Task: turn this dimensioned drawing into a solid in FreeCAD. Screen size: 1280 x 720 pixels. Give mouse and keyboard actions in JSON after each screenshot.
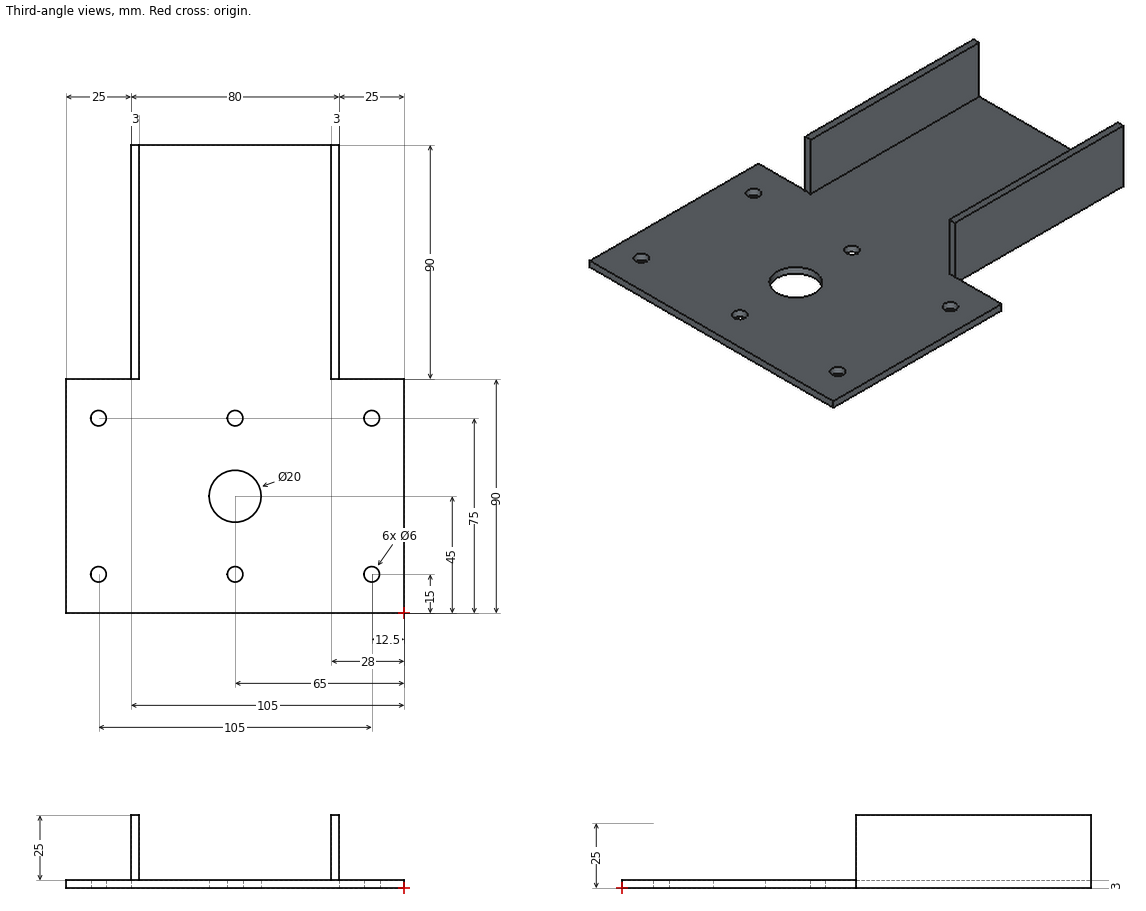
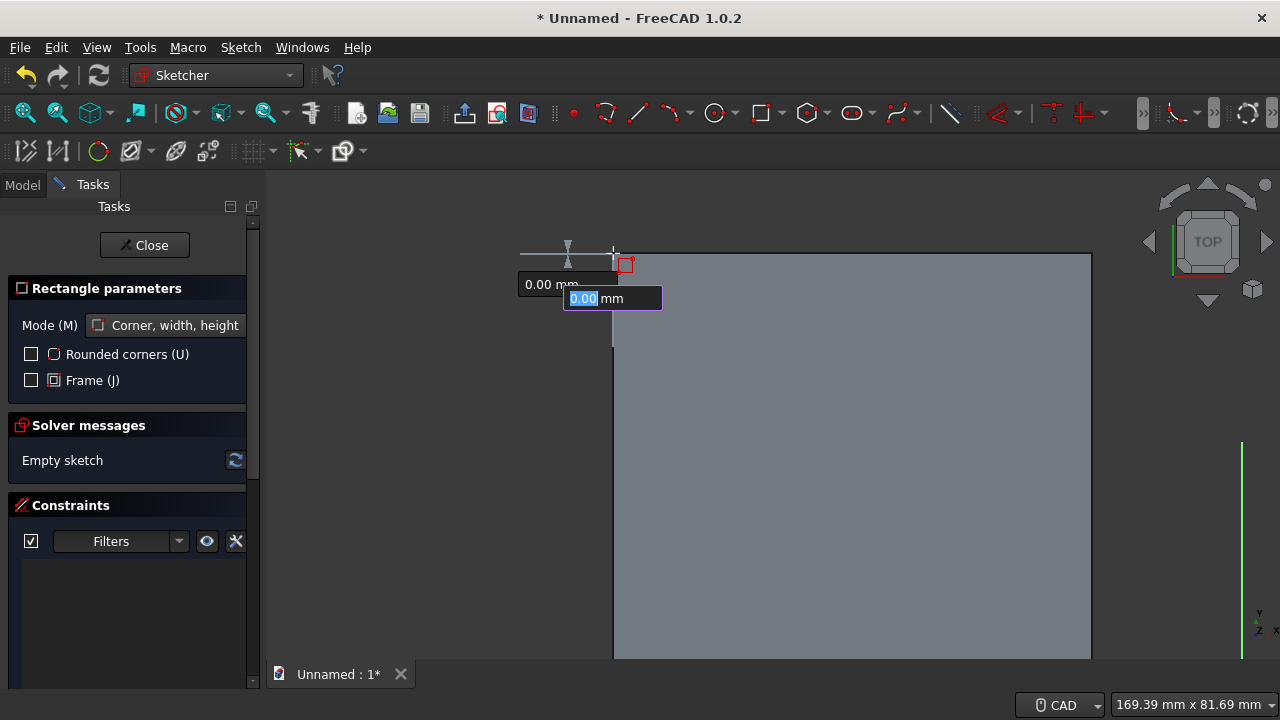
{"action": "scroll", "coordinate": [608, 252], "scroll_direction": "down", "scroll_amount": 6}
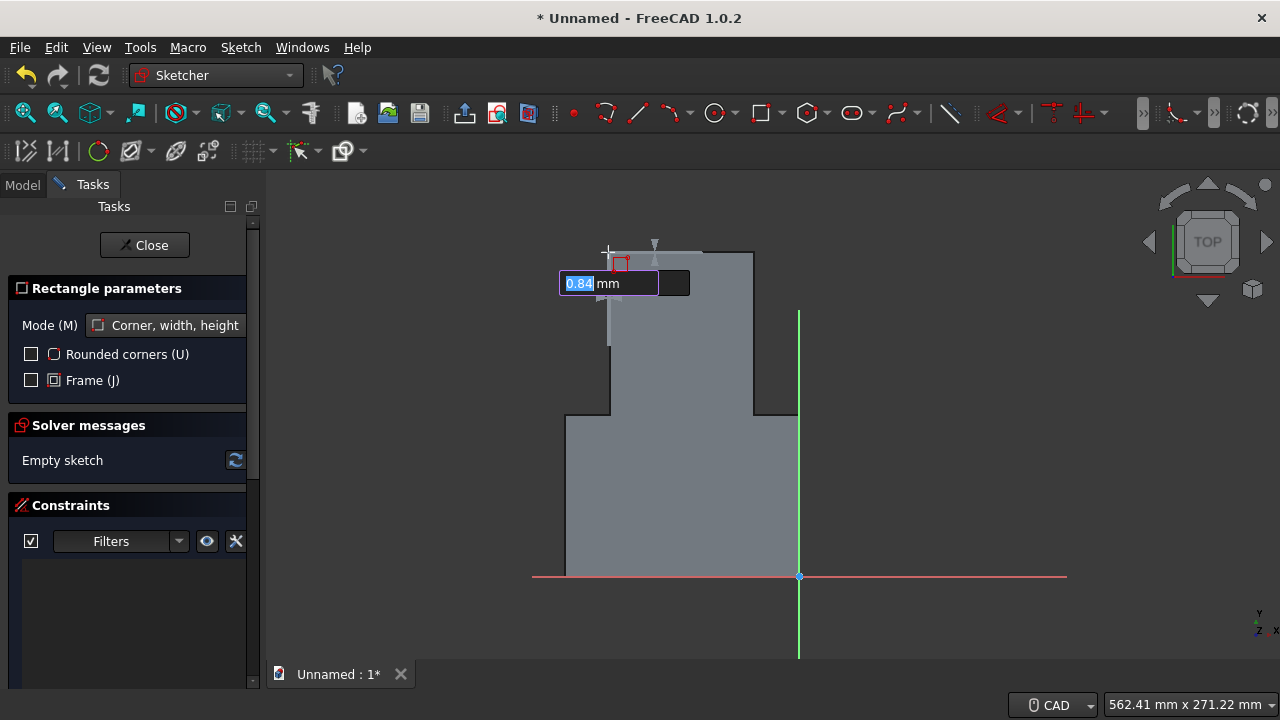
{"action": "left_click", "coordinate": [615, 415]}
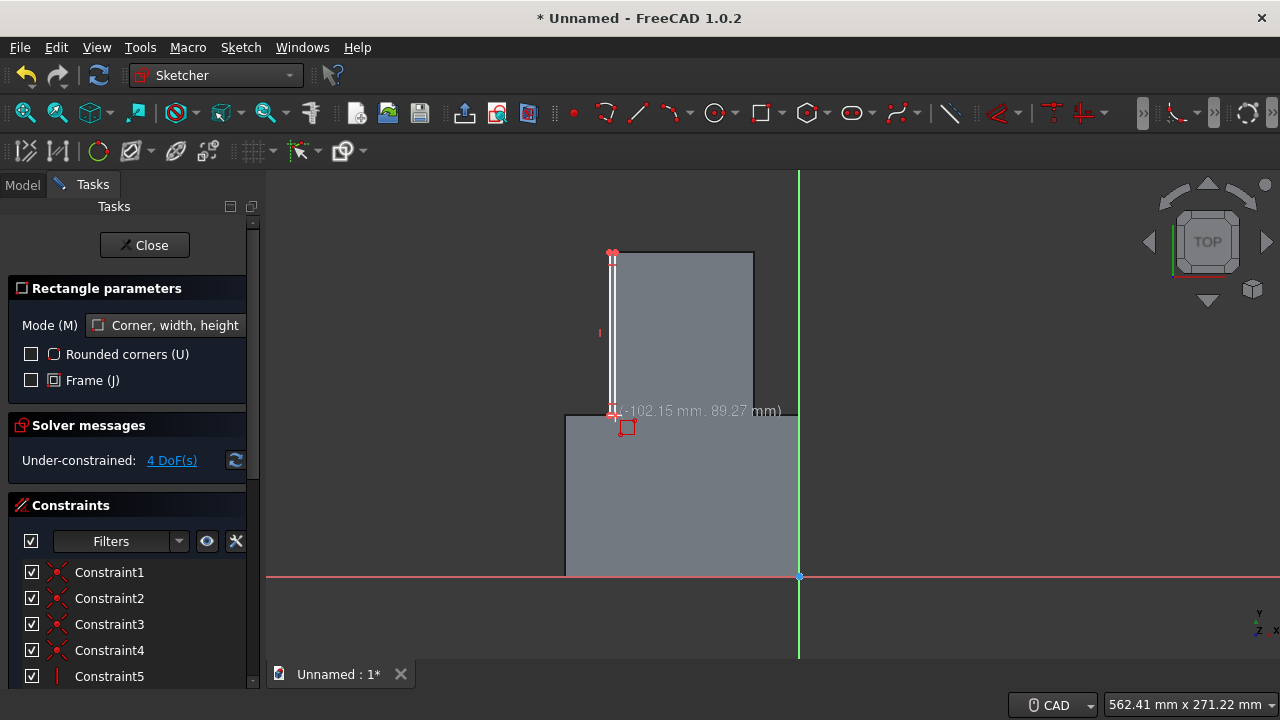
{"action": "scroll", "coordinate": [749, 252], "scroll_direction": "up", "scroll_amount": 6}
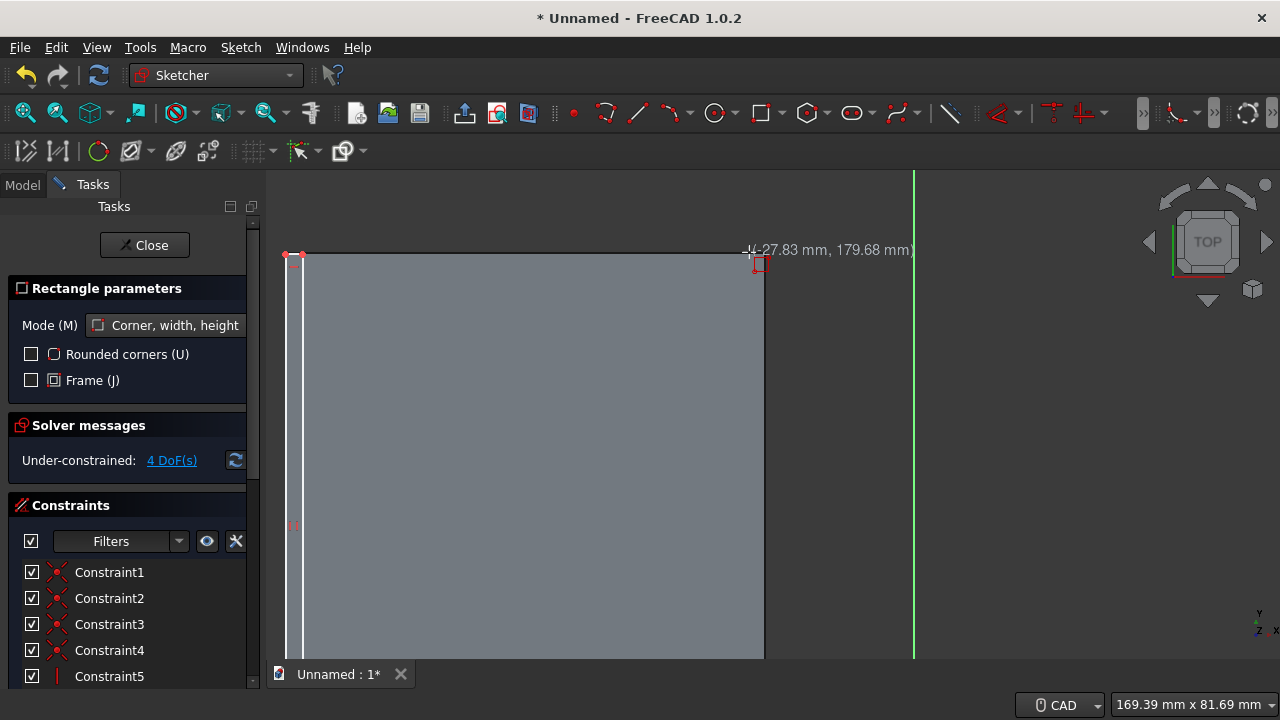
{"action": "left_click", "coordinate": [747, 253]}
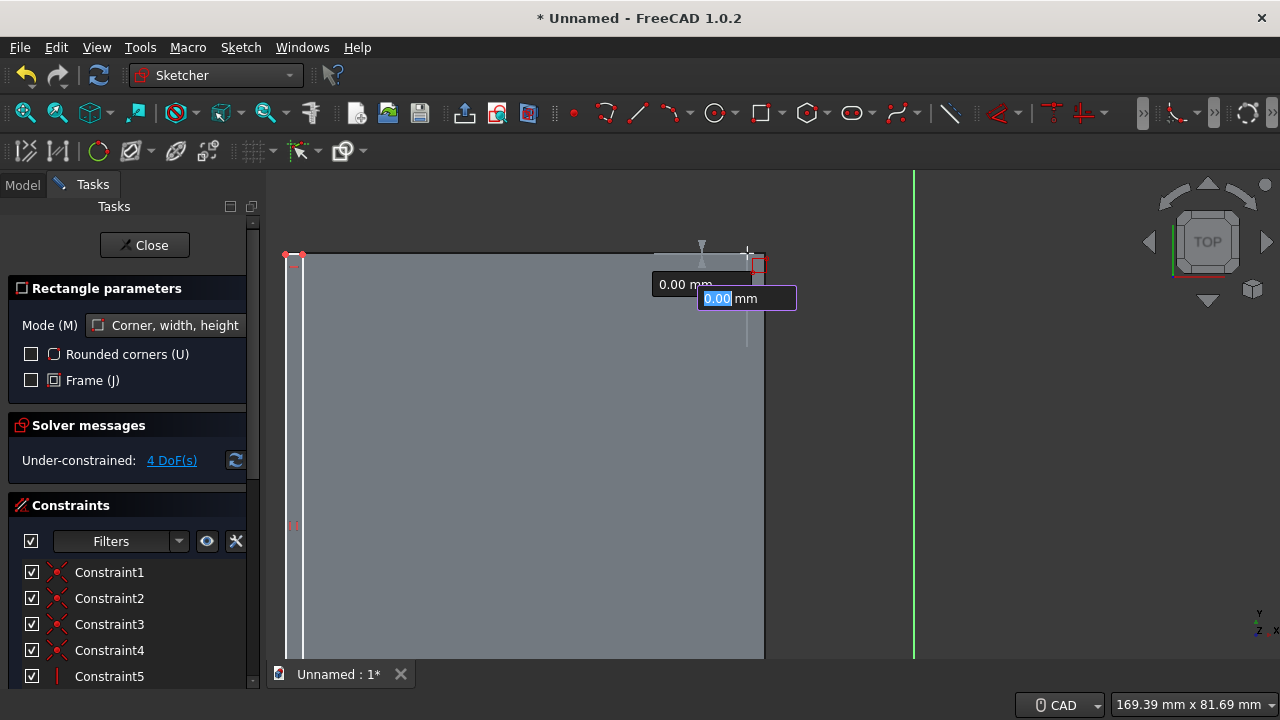
{"action": "scroll", "coordinate": [749, 252], "scroll_direction": "down", "scroll_amount": 6}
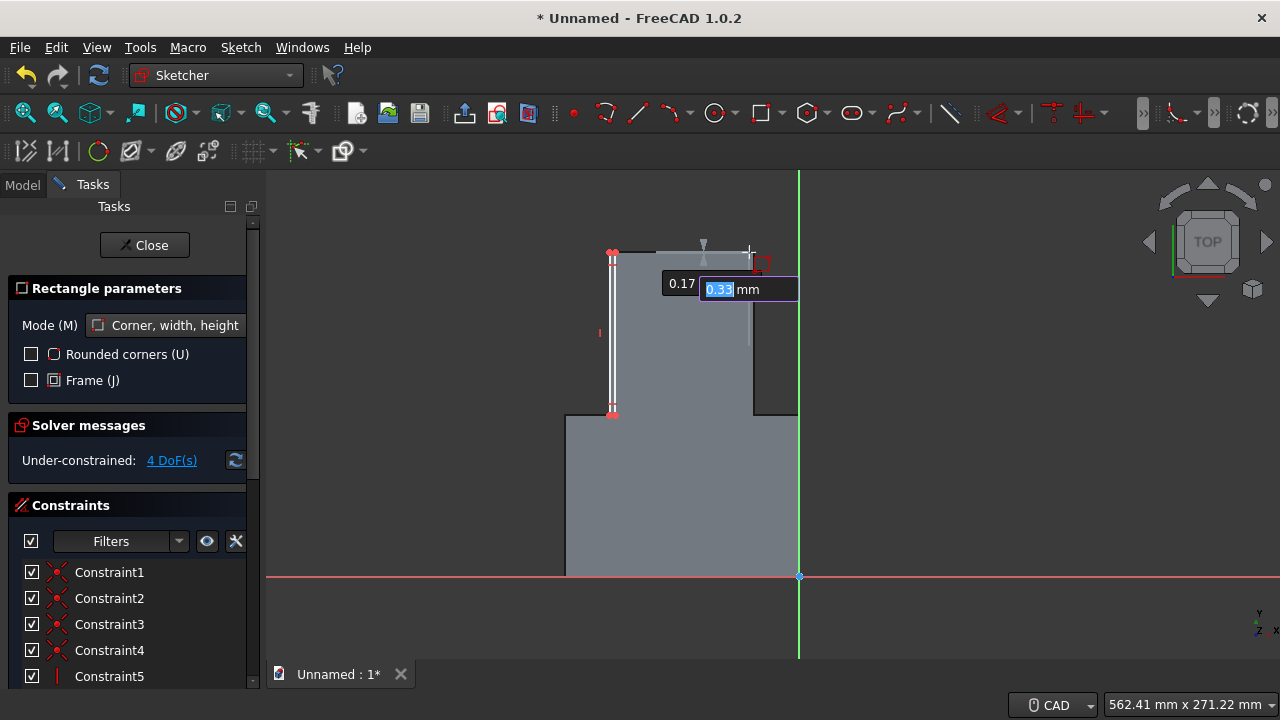
{"action": "left_click", "coordinate": [754, 415]}
{"action": "key", "text": "Escape"}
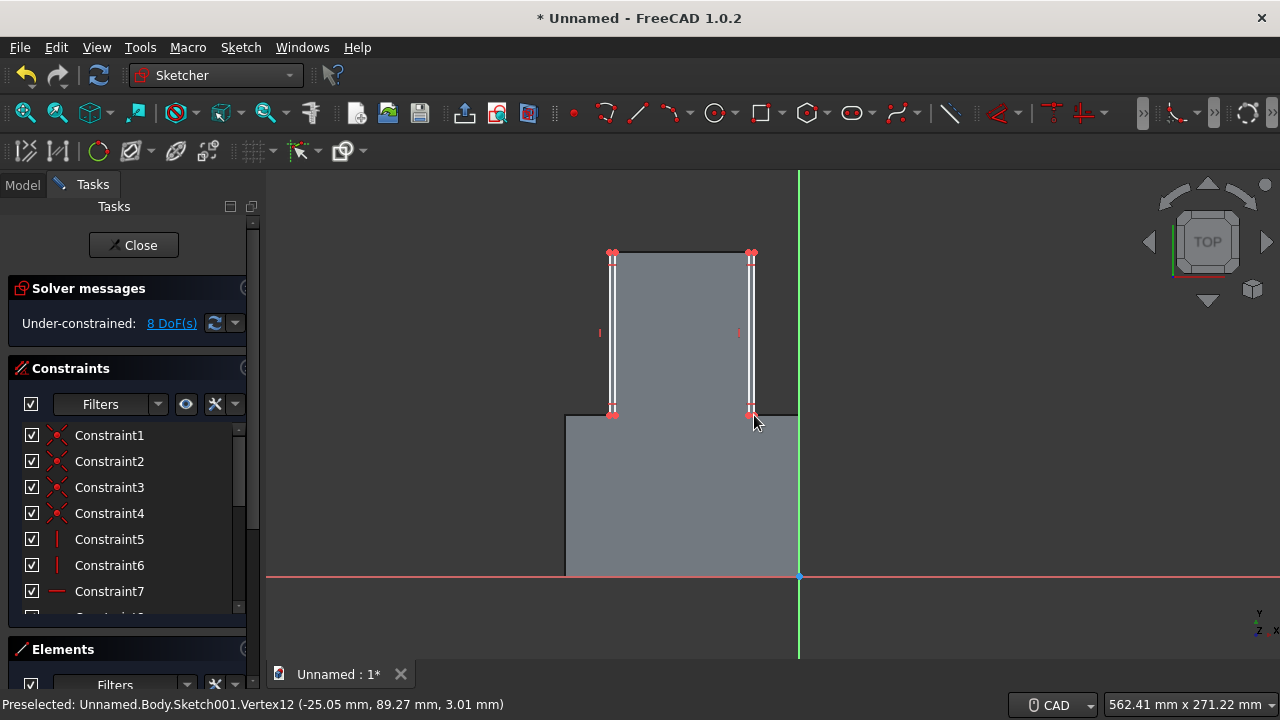
{"action": "left_click", "coordinate": [998, 114]}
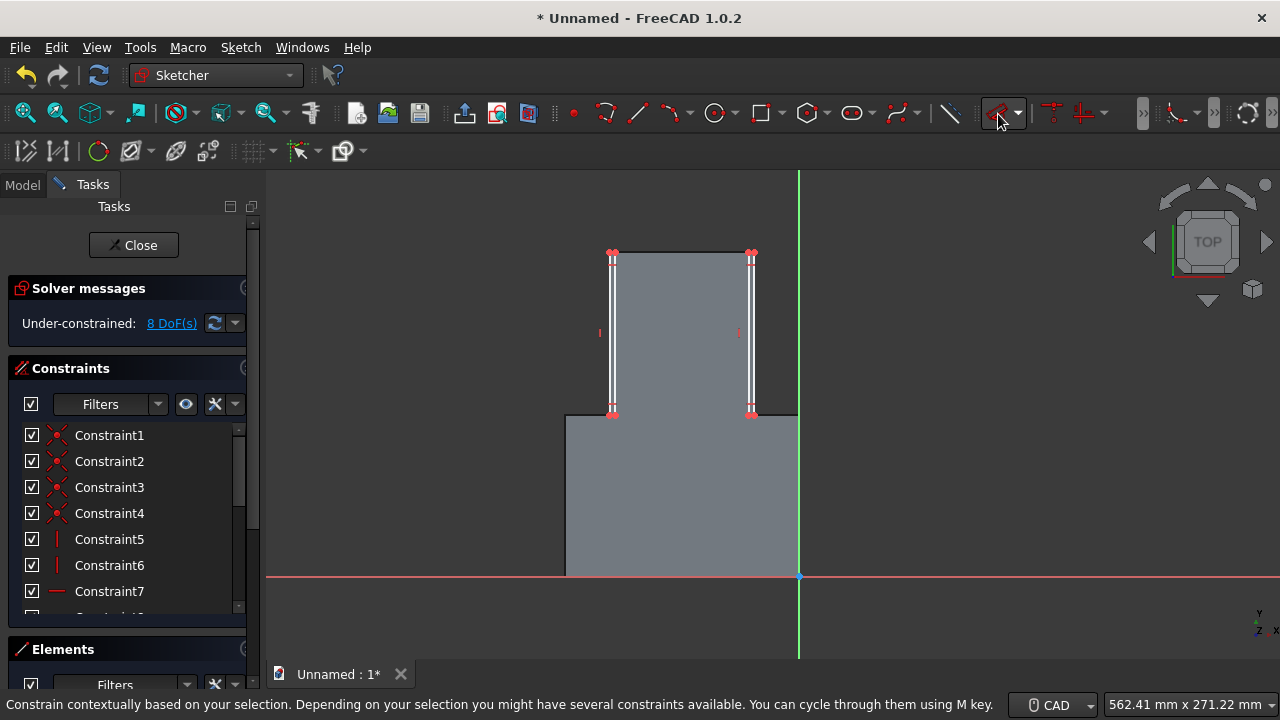
{"action": "scroll", "coordinate": [612, 416], "scroll_direction": "up", "scroll_amount": 10}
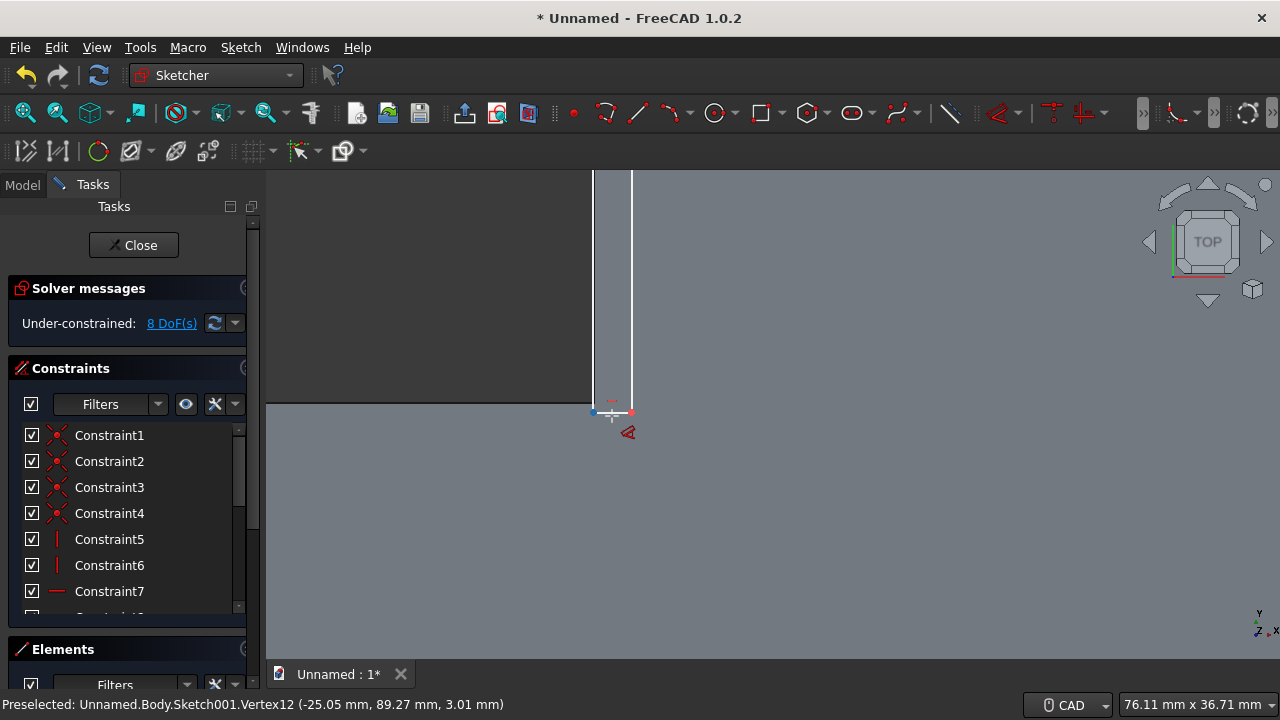
{"action": "left_click", "coordinate": [613, 413]}
{"action": "left_click", "coordinate": [613, 447]}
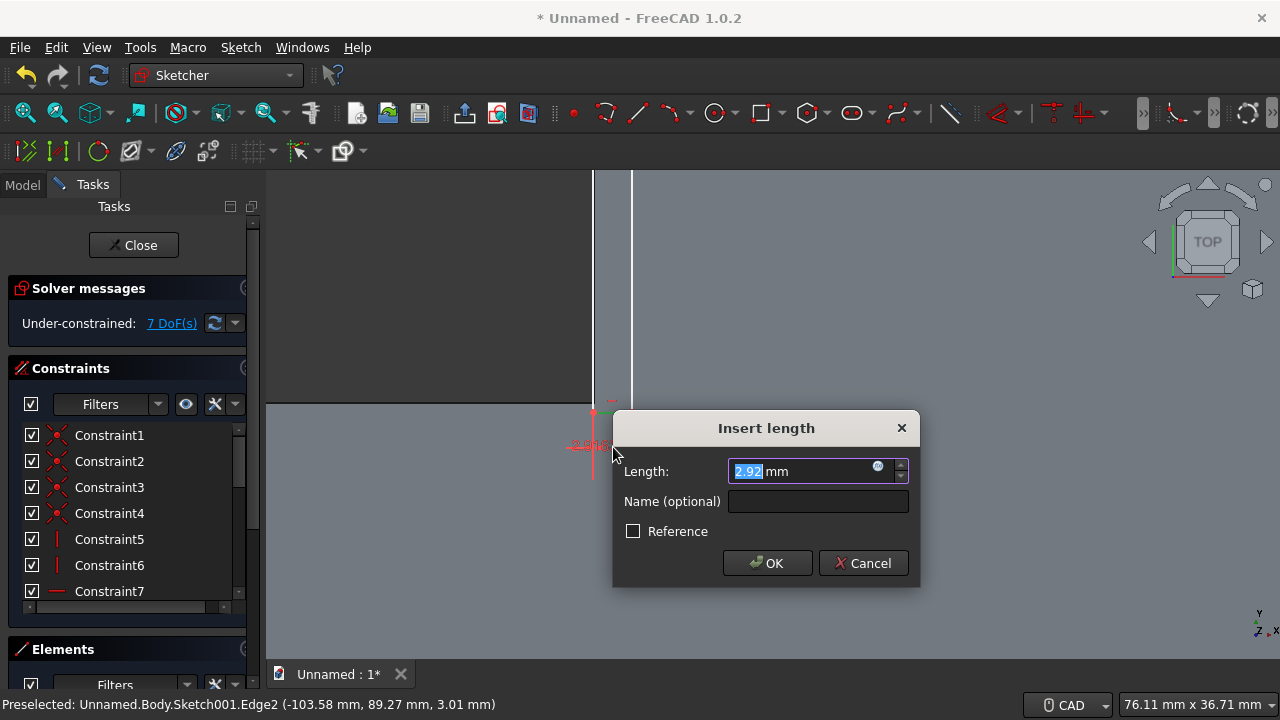
{"action": "type", "text": "3"}
{"action": "key", "text": "Return"}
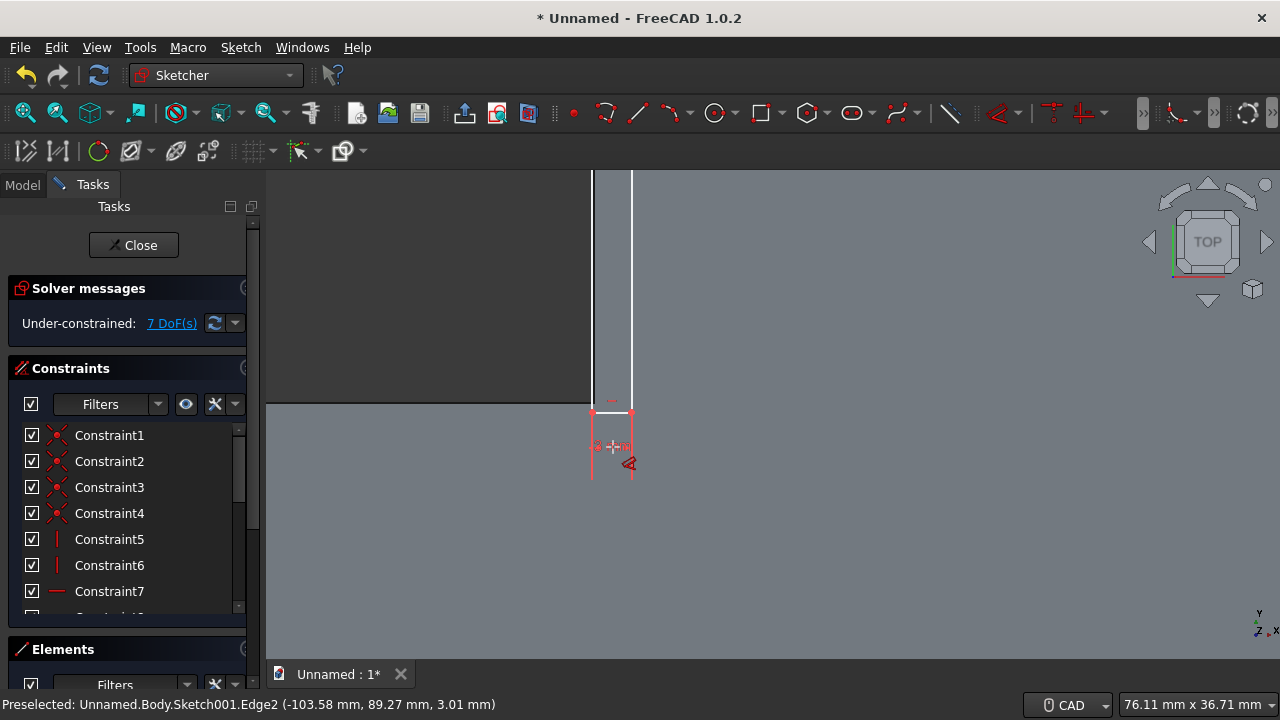
{"action": "scroll", "coordinate": [612, 416], "scroll_direction": "down", "scroll_amount": 10}